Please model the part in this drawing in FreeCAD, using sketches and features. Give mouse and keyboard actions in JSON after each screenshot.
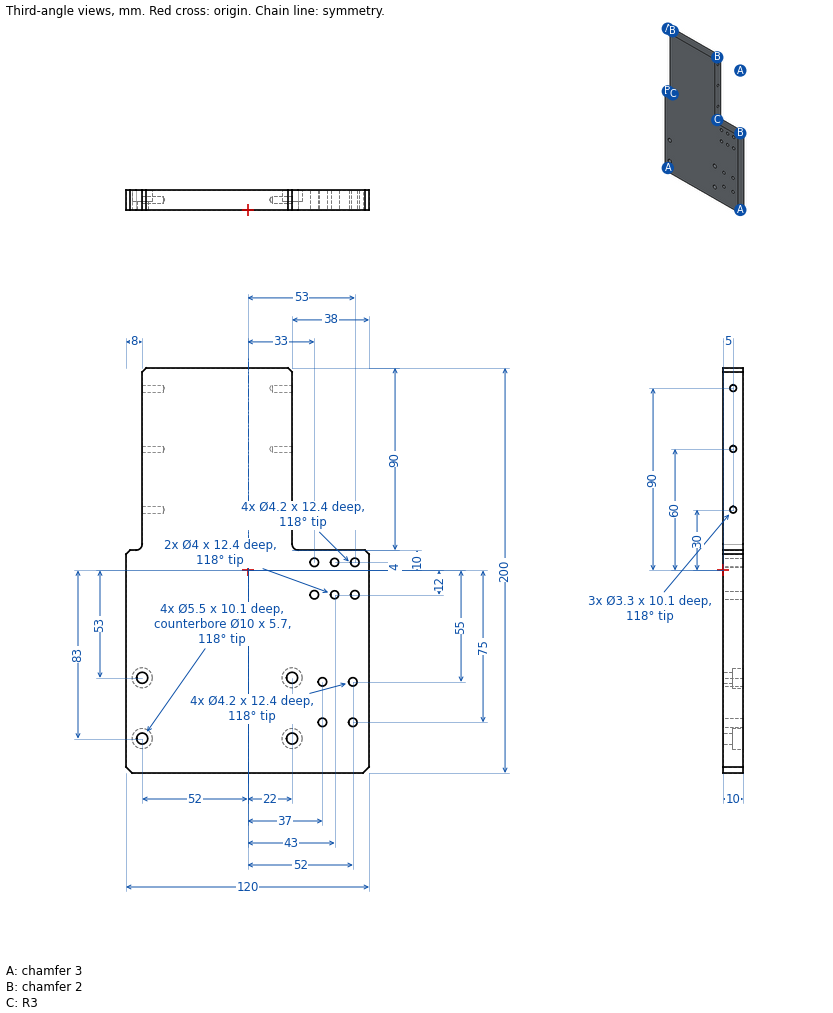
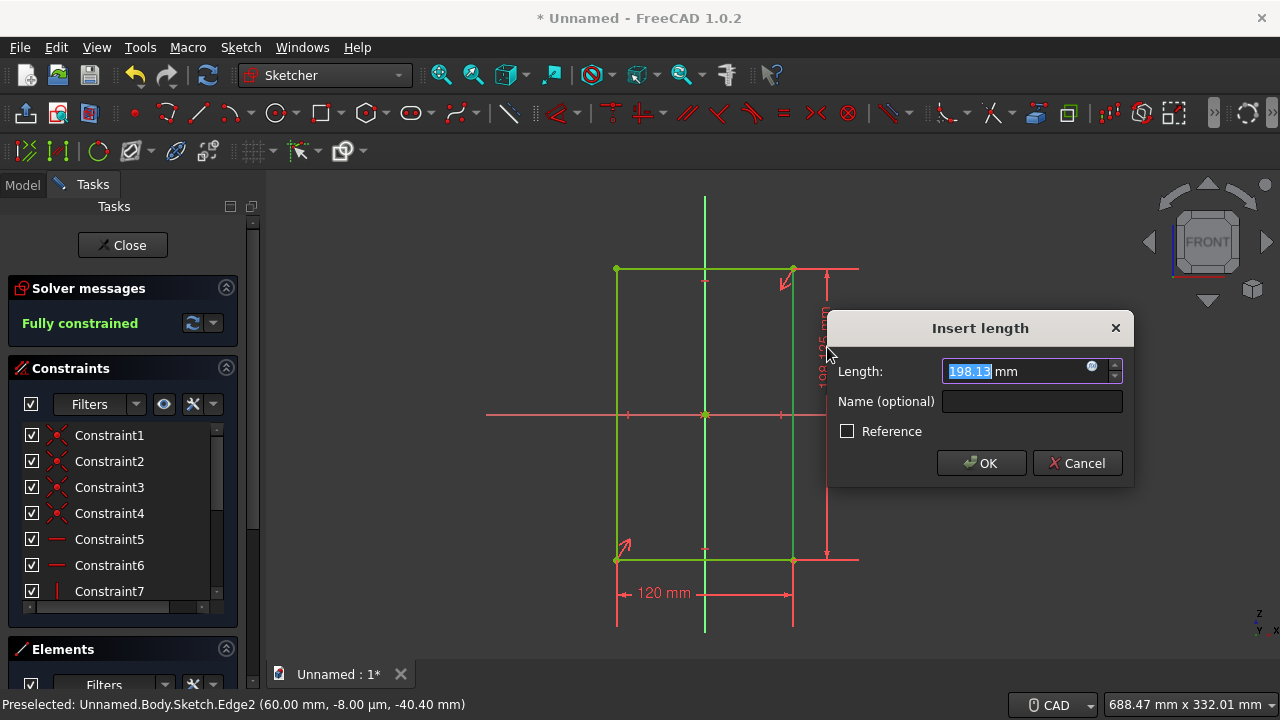
{"action": "type", "text": "200"}
{"action": "key", "text": "Return"}
{"action": "key", "text": "Escape"}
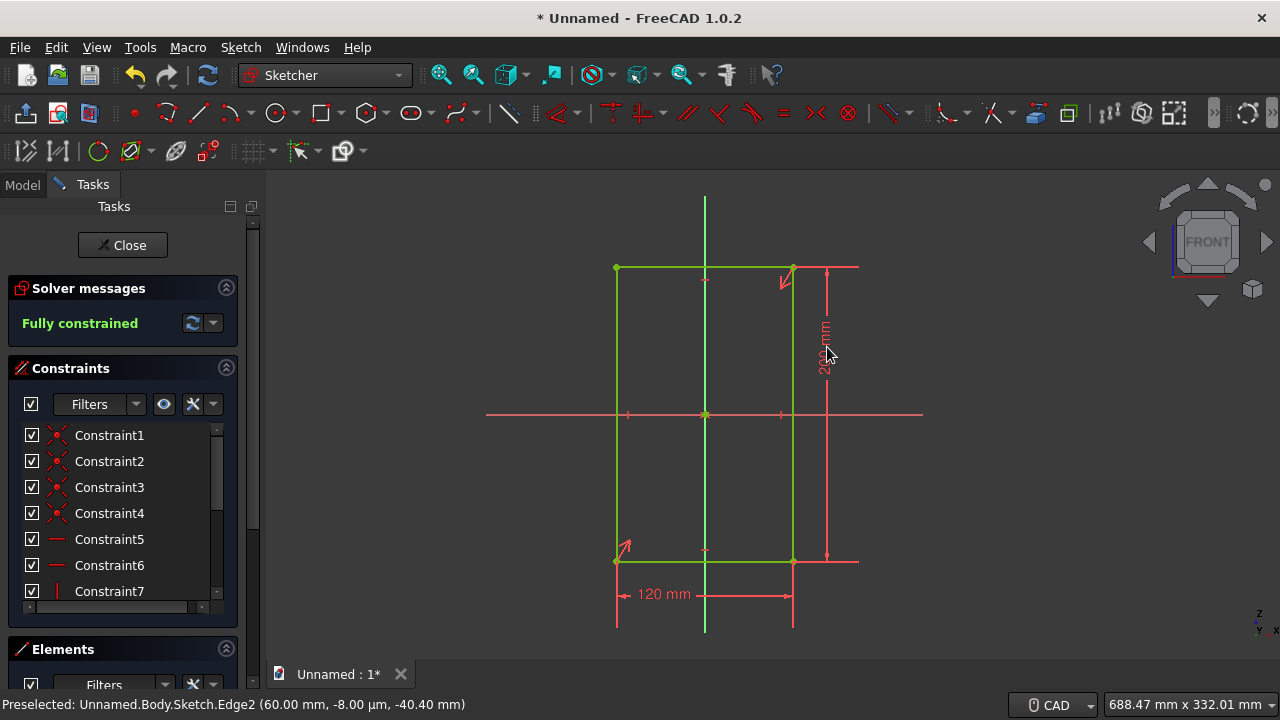
{"action": "left_click", "coordinate": [123, 245]}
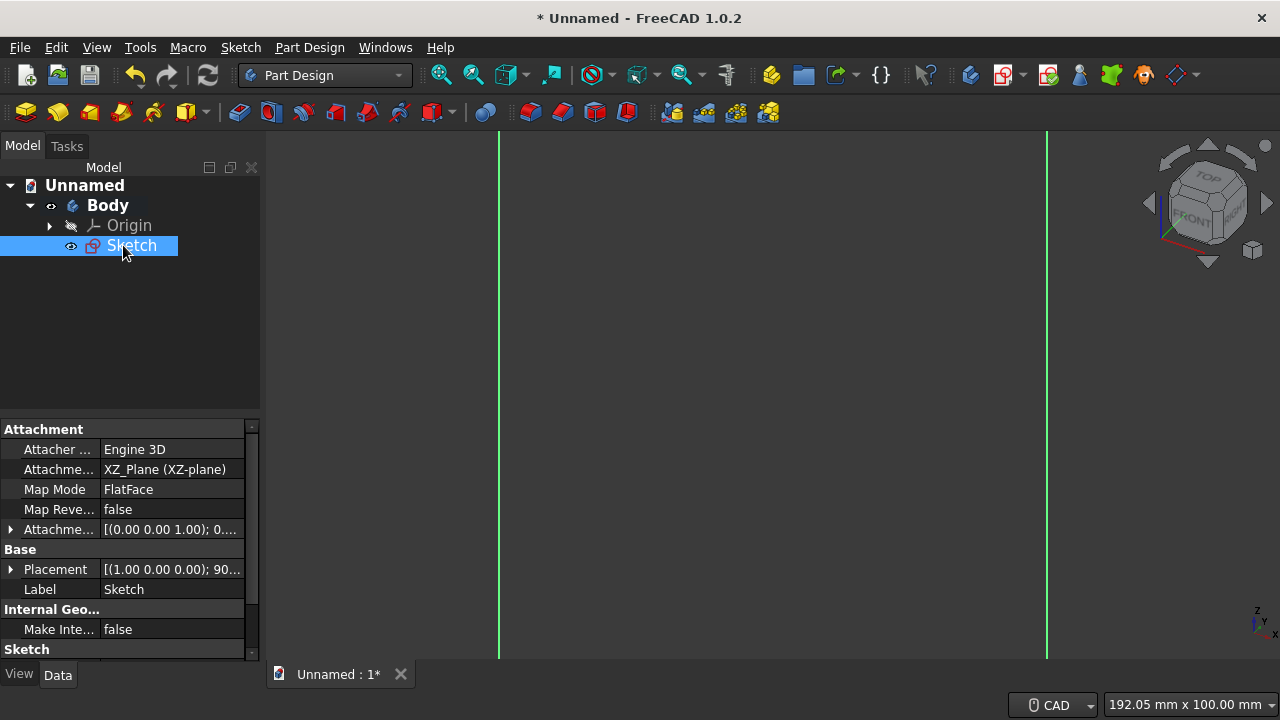
{"action": "left_click", "coordinate": [26, 112]}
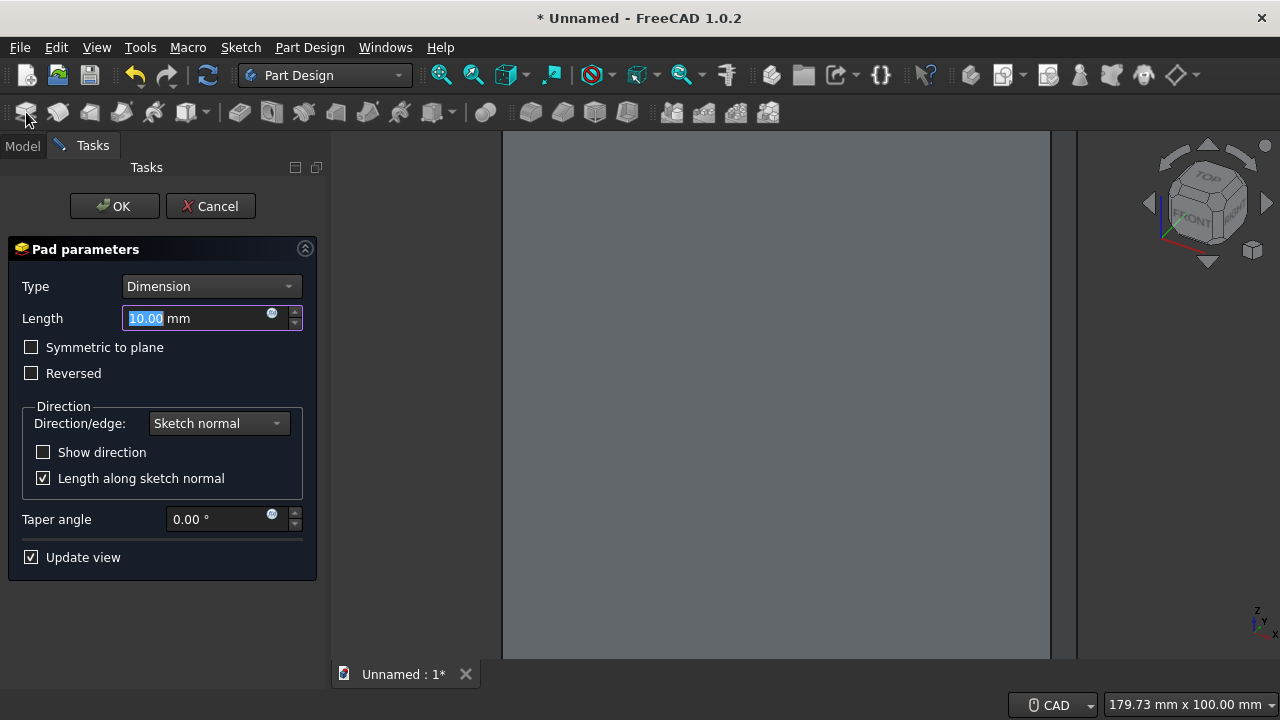
{"action": "type", "text": "10"}
{"action": "key", "text": "Tab"}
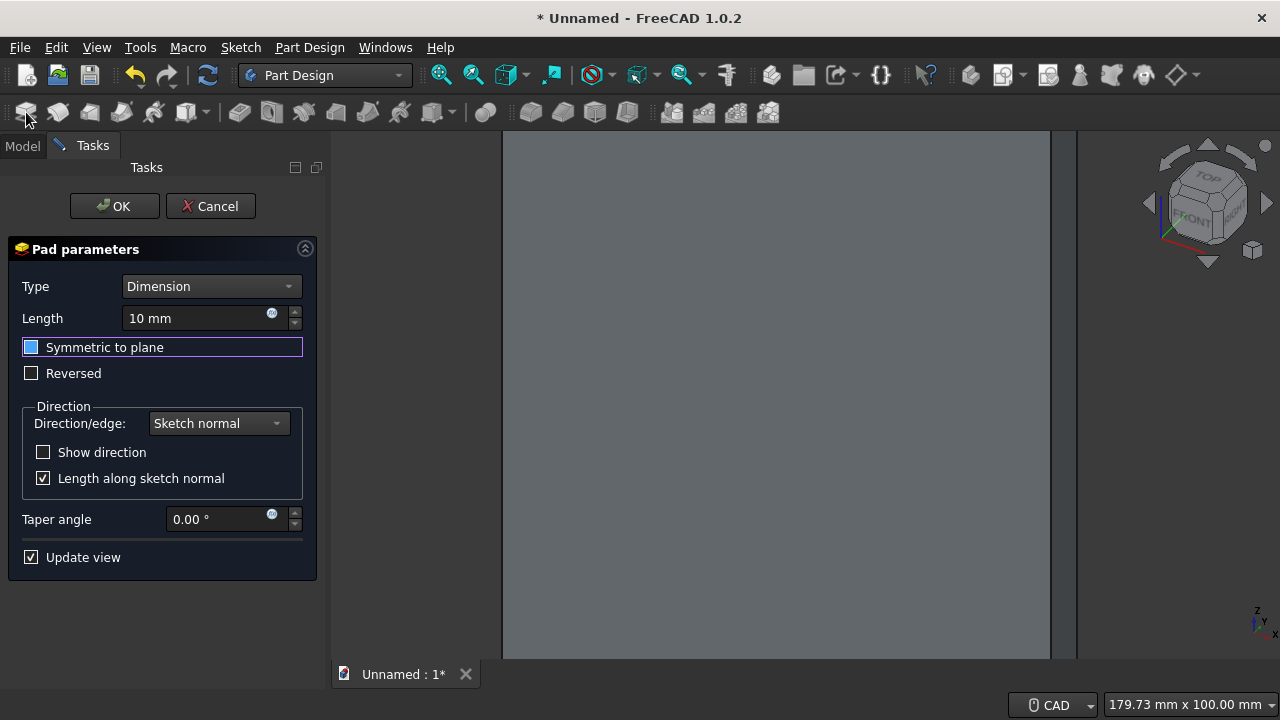
{"action": "left_click", "coordinate": [30, 373]}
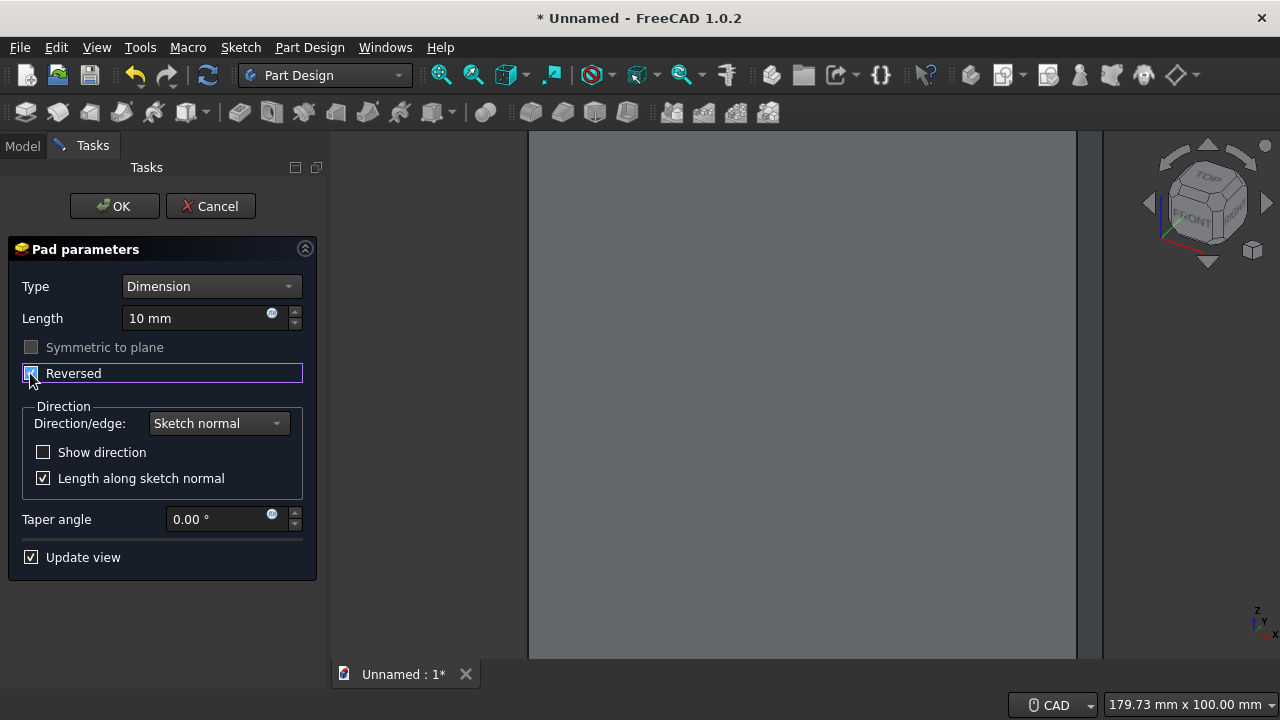
{"action": "left_click", "coordinate": [115, 206]}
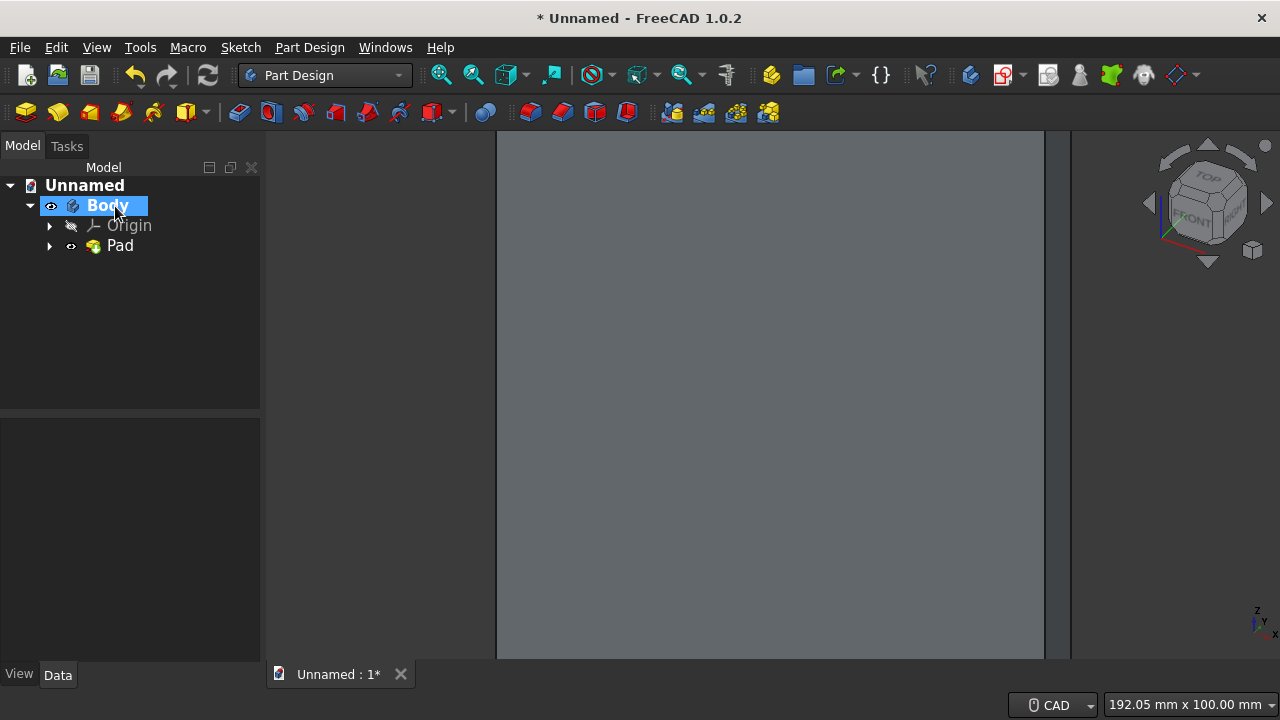
{"action": "left_click", "coordinate": [442, 76]}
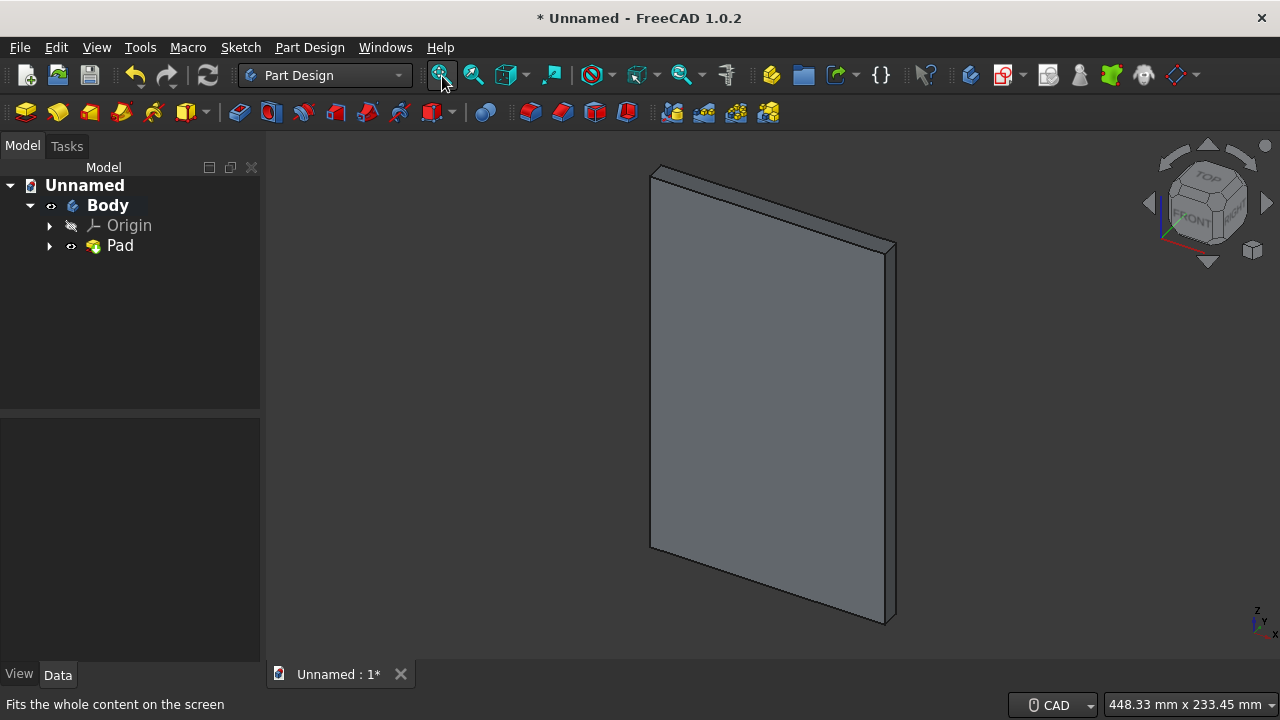
{"action": "left_click", "coordinate": [891, 248]}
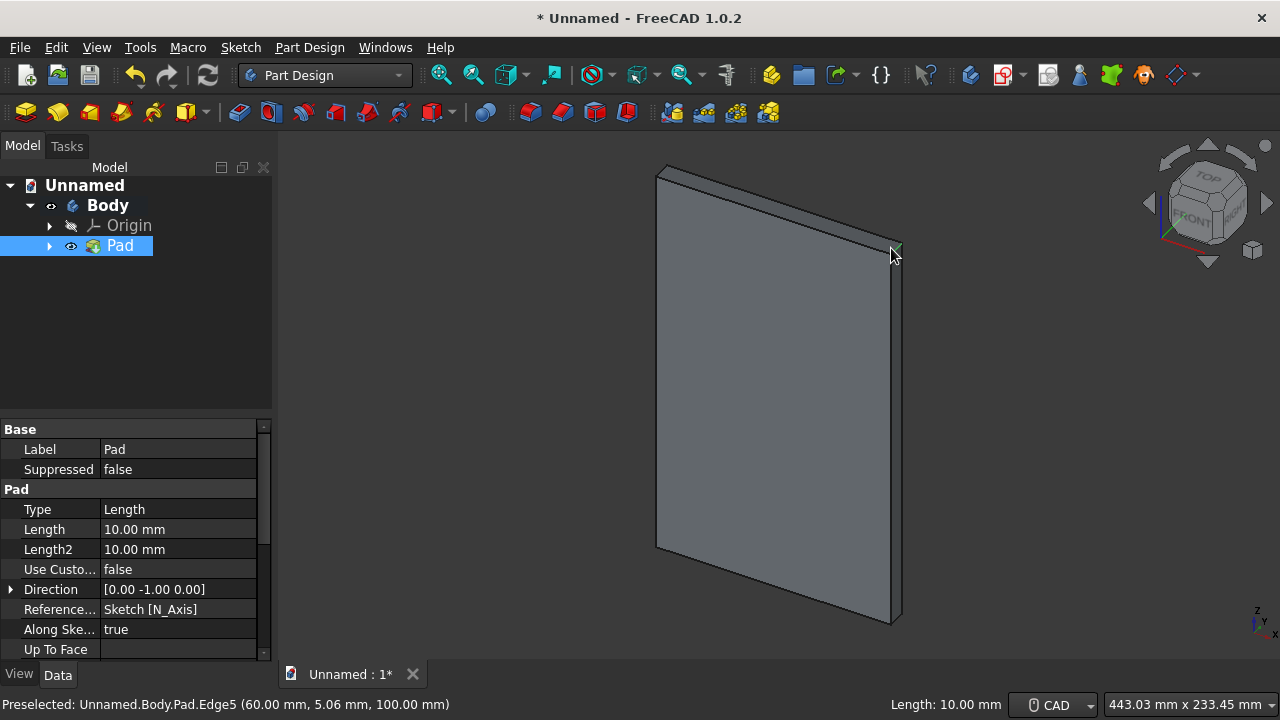
{"action": "key", "text": "0"}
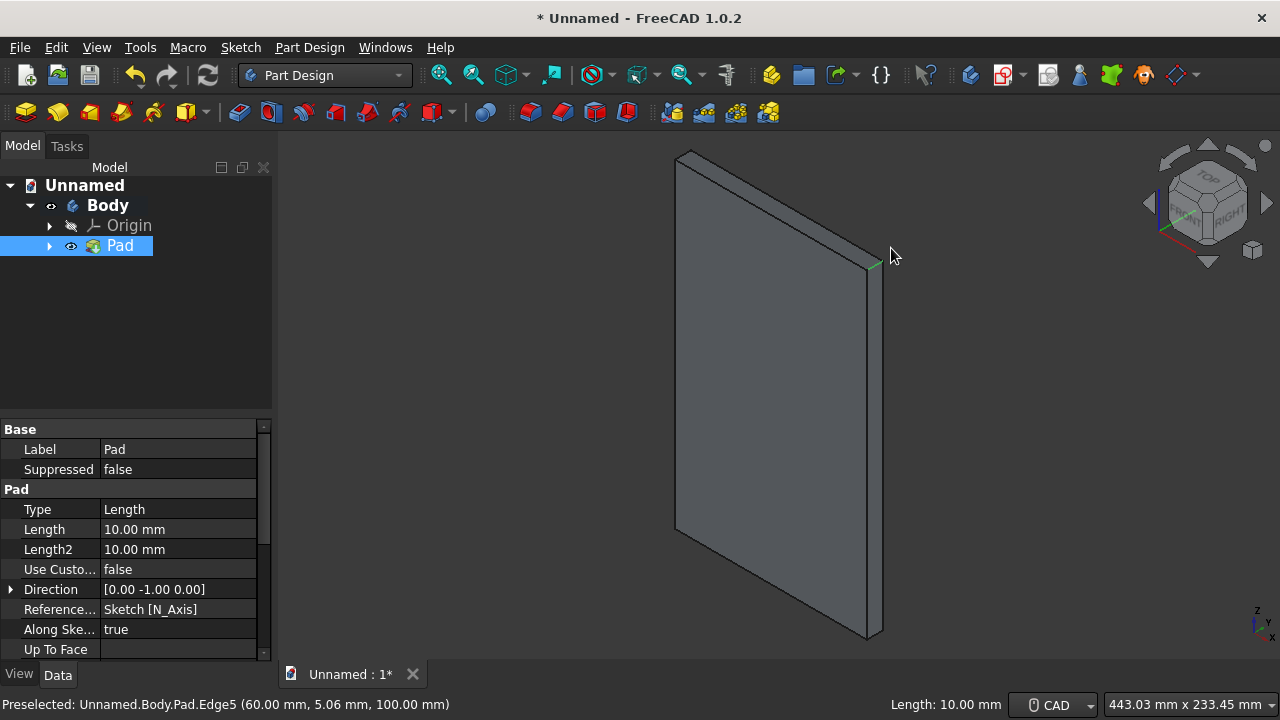
{"action": "key", "text": "2"}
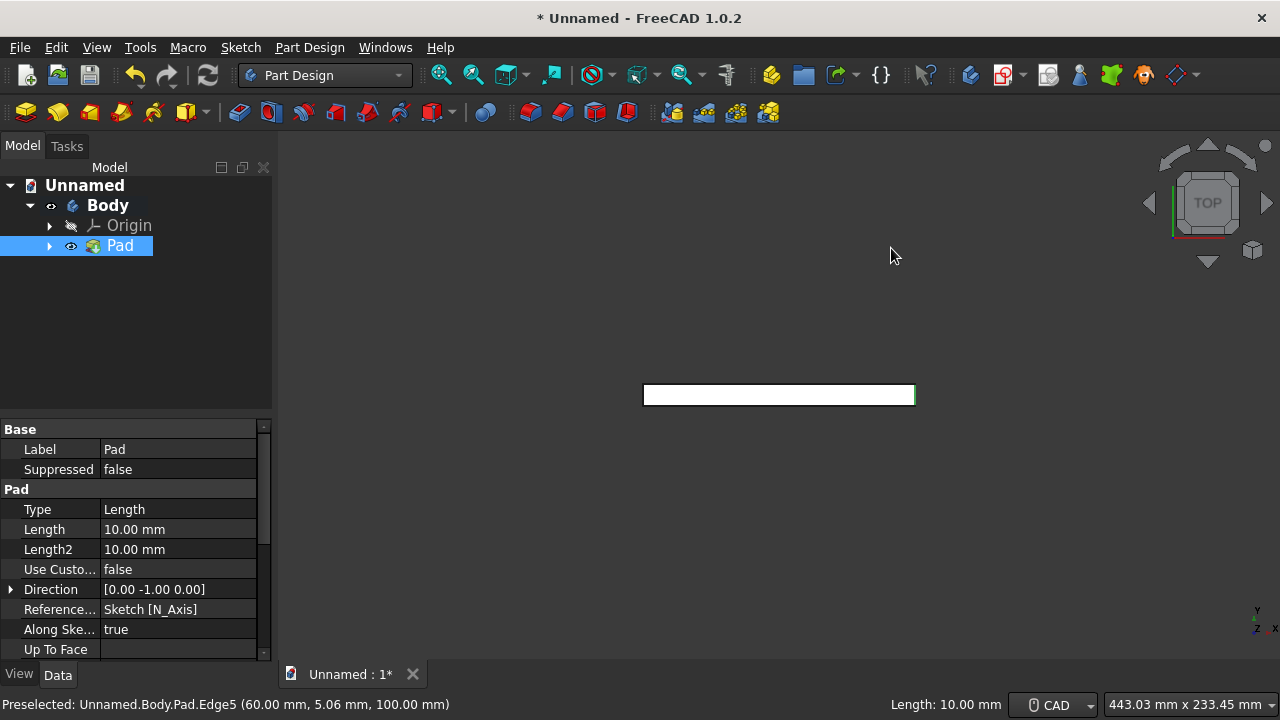
{"action": "key", "text": "v f"}